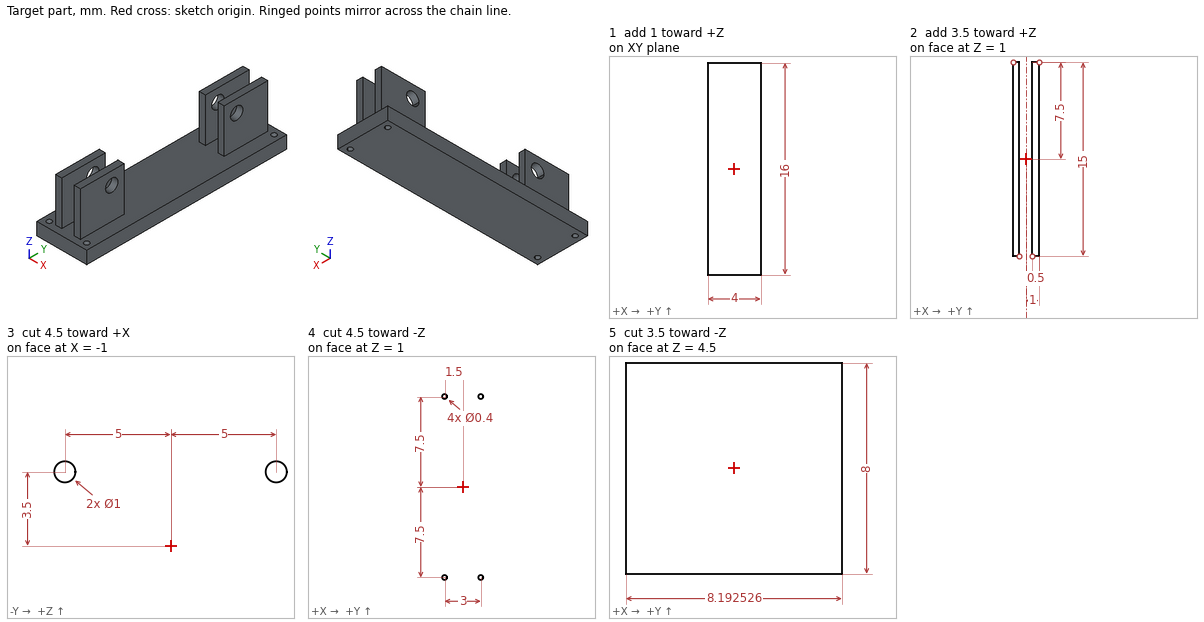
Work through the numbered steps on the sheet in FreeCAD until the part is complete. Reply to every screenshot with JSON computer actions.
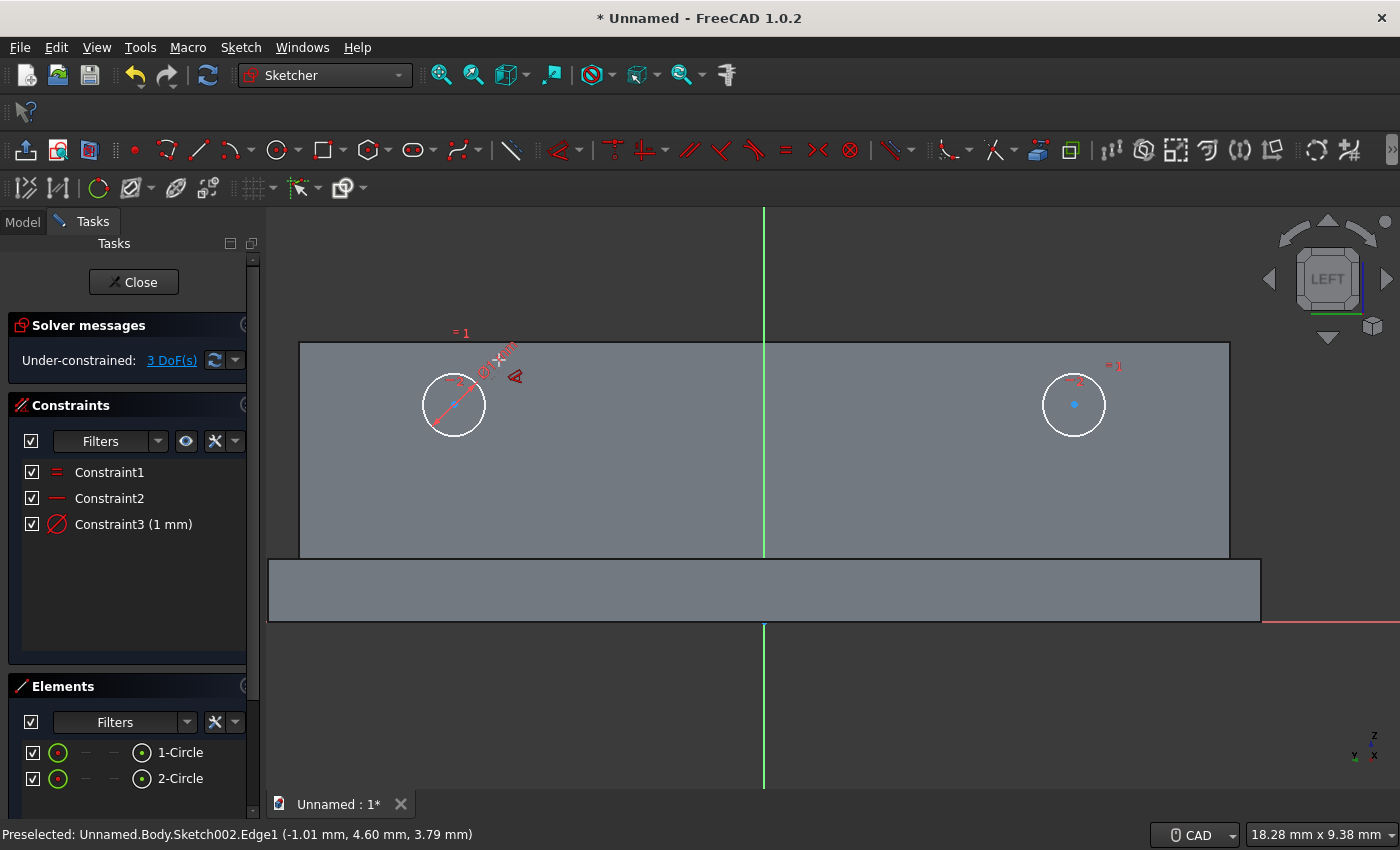
{"action": "left_click", "coordinate": [454, 405]}
{"action": "left_click", "coordinate": [609, 656]}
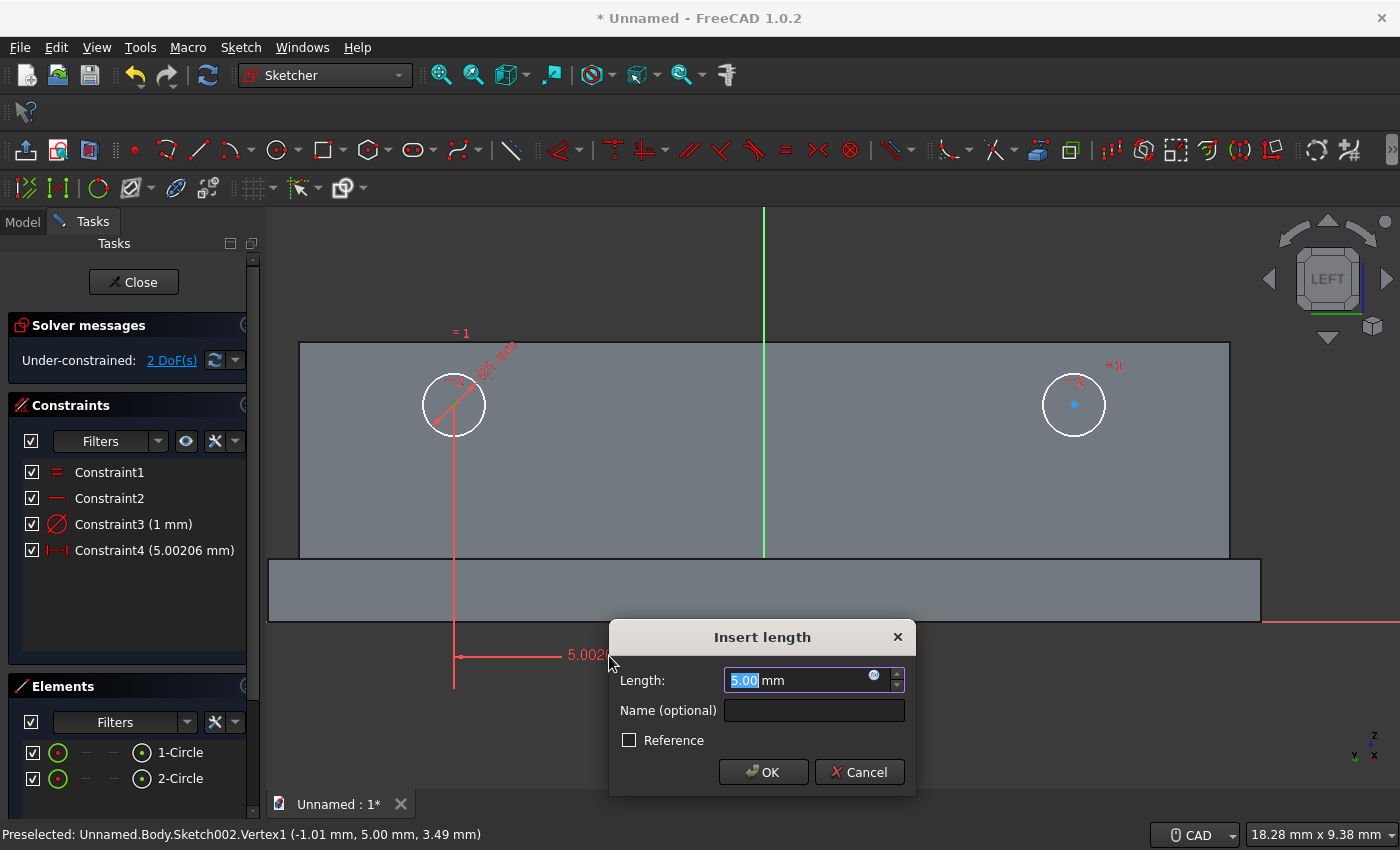
{"action": "type", "text": "5"}
{"action": "key", "text": "Return"}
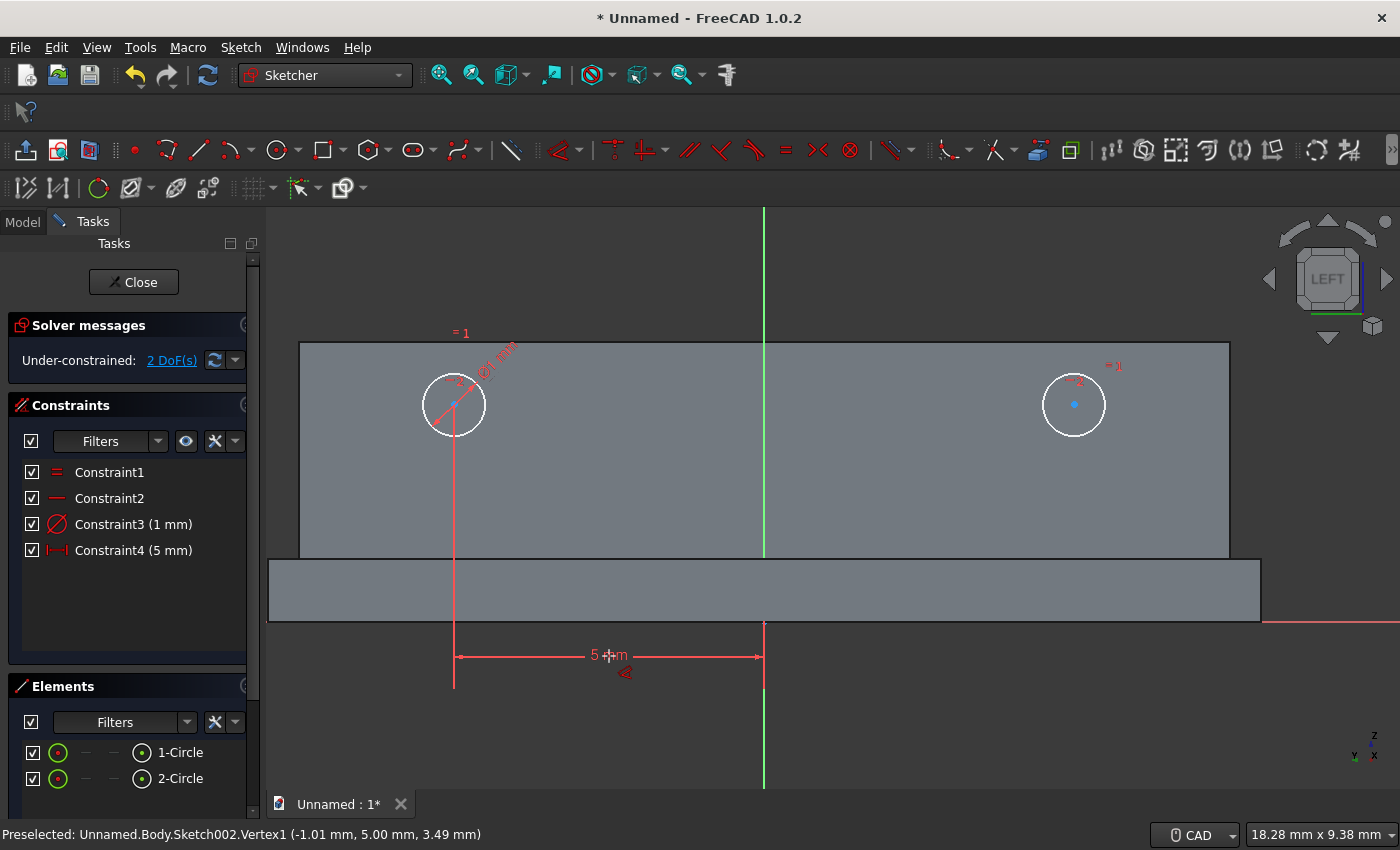
{"action": "left_click", "coordinate": [1074, 405]}
{"action": "left_click", "coordinate": [919, 656]}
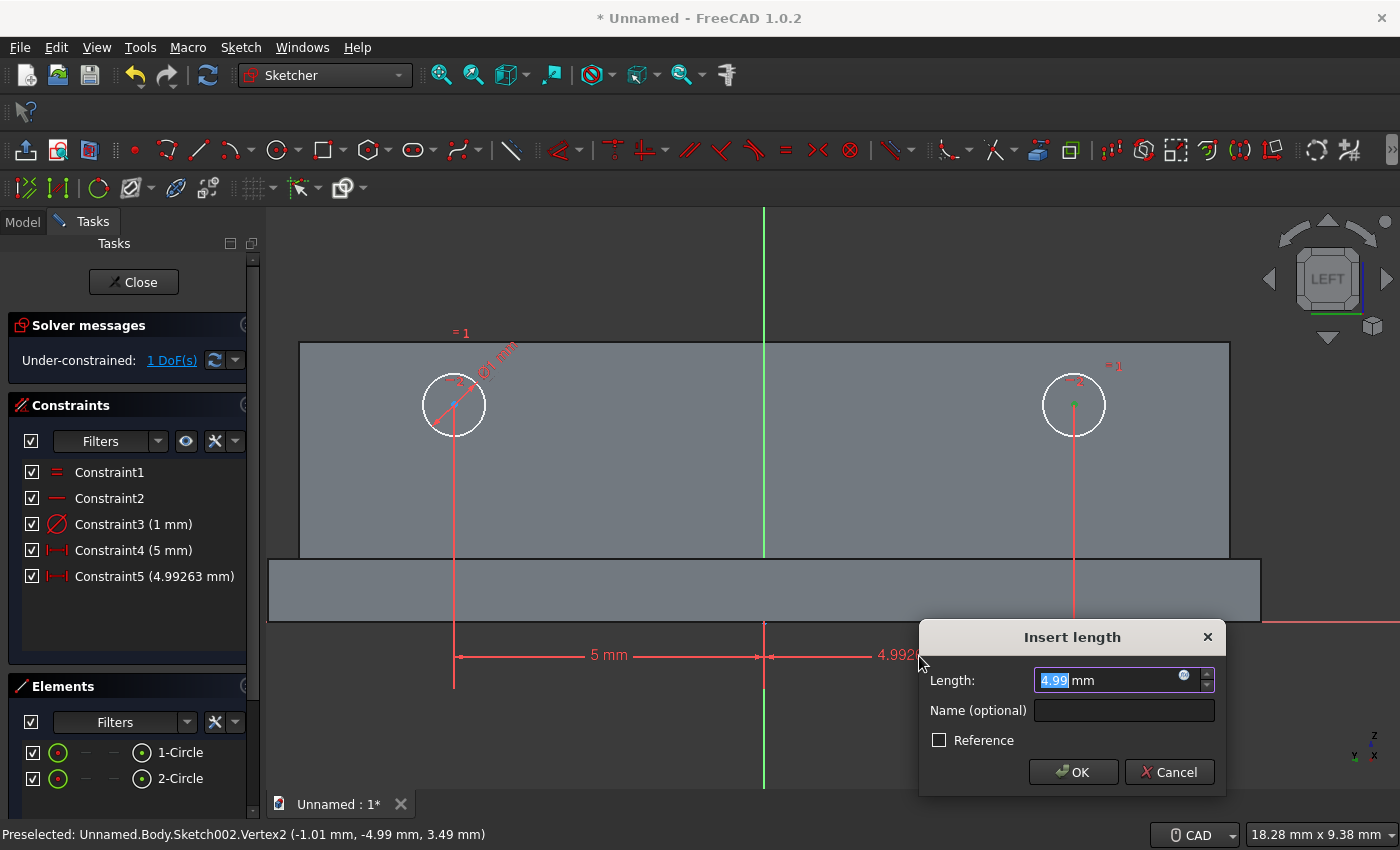
{"action": "type", "text": "5"}
{"action": "key", "text": "Return"}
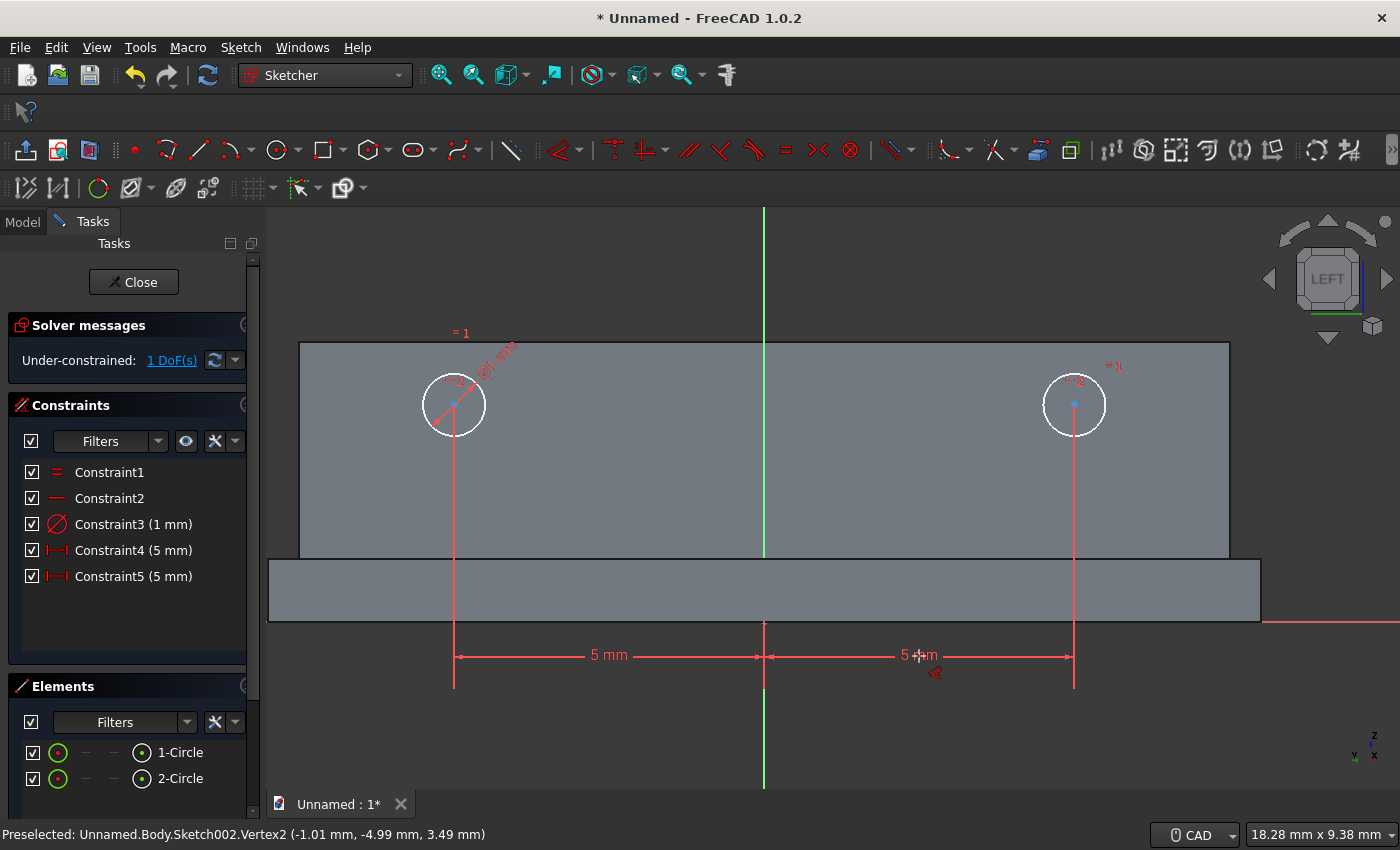
{"action": "left_click", "coordinate": [454, 405]}
{"action": "left_click", "coordinate": [420, 513]}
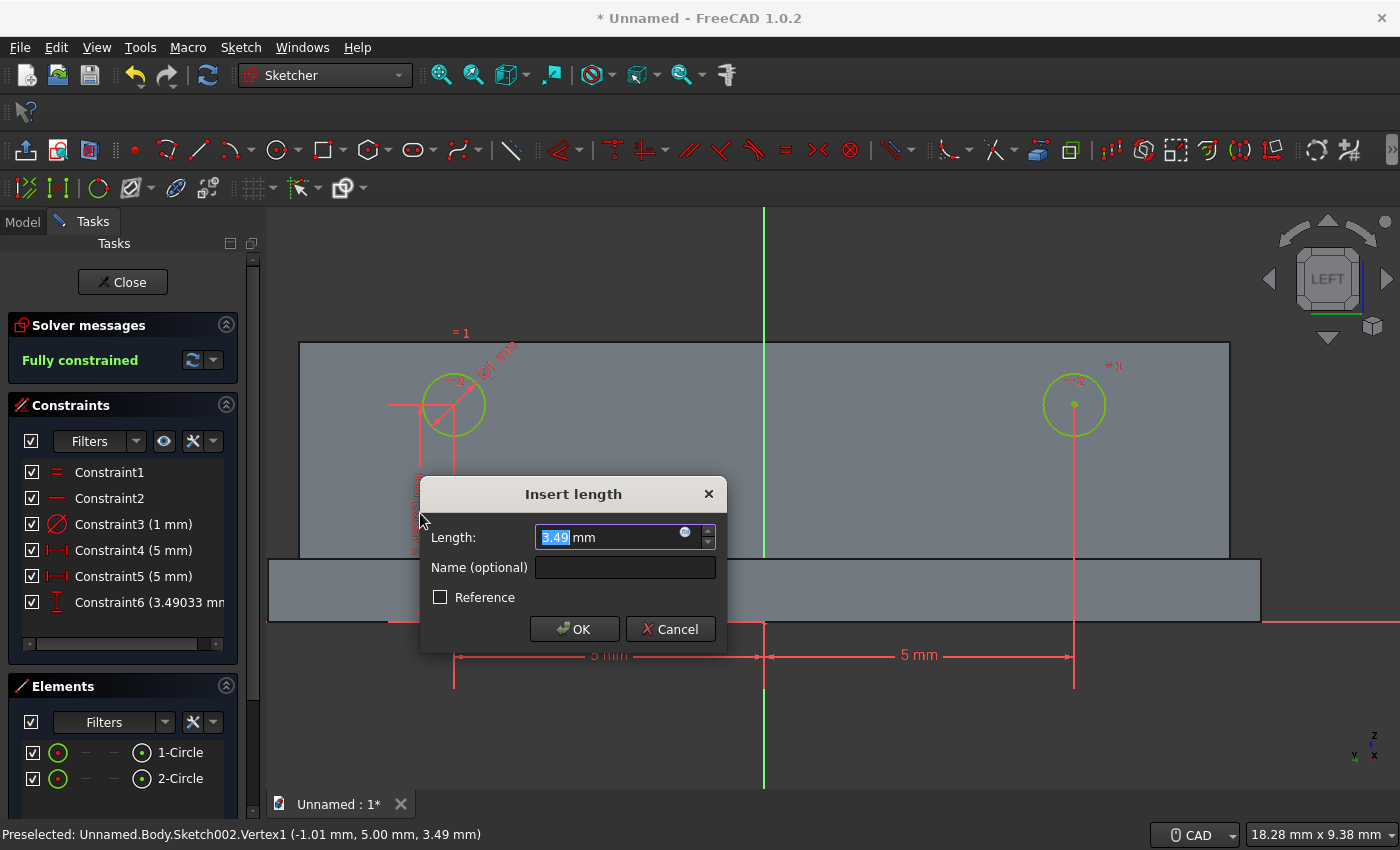
{"action": "type", "text": "3.5"}
{"action": "key", "text": "Return"}
{"action": "key", "text": "Escape"}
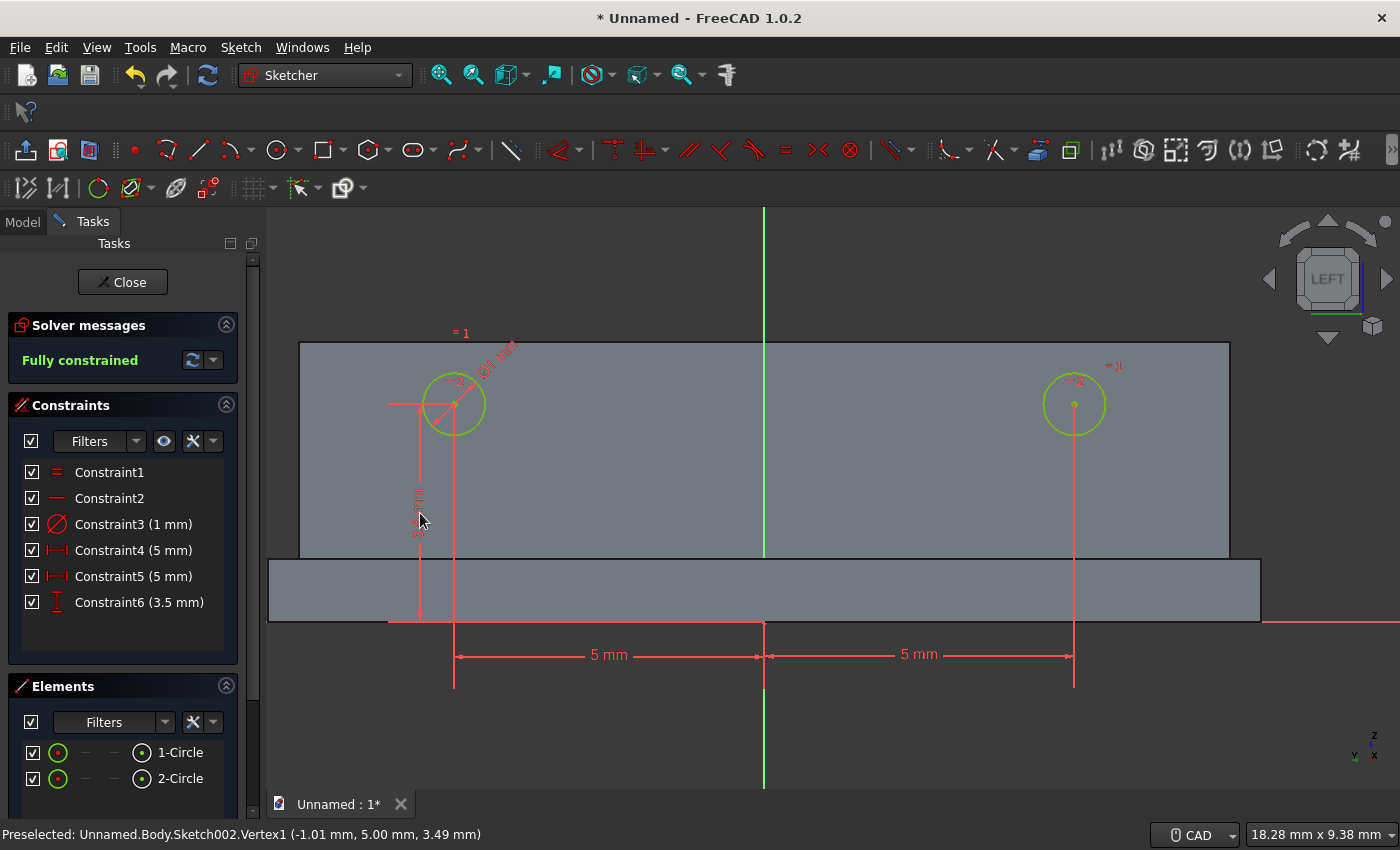
{"action": "left_click", "coordinate": [123, 282]}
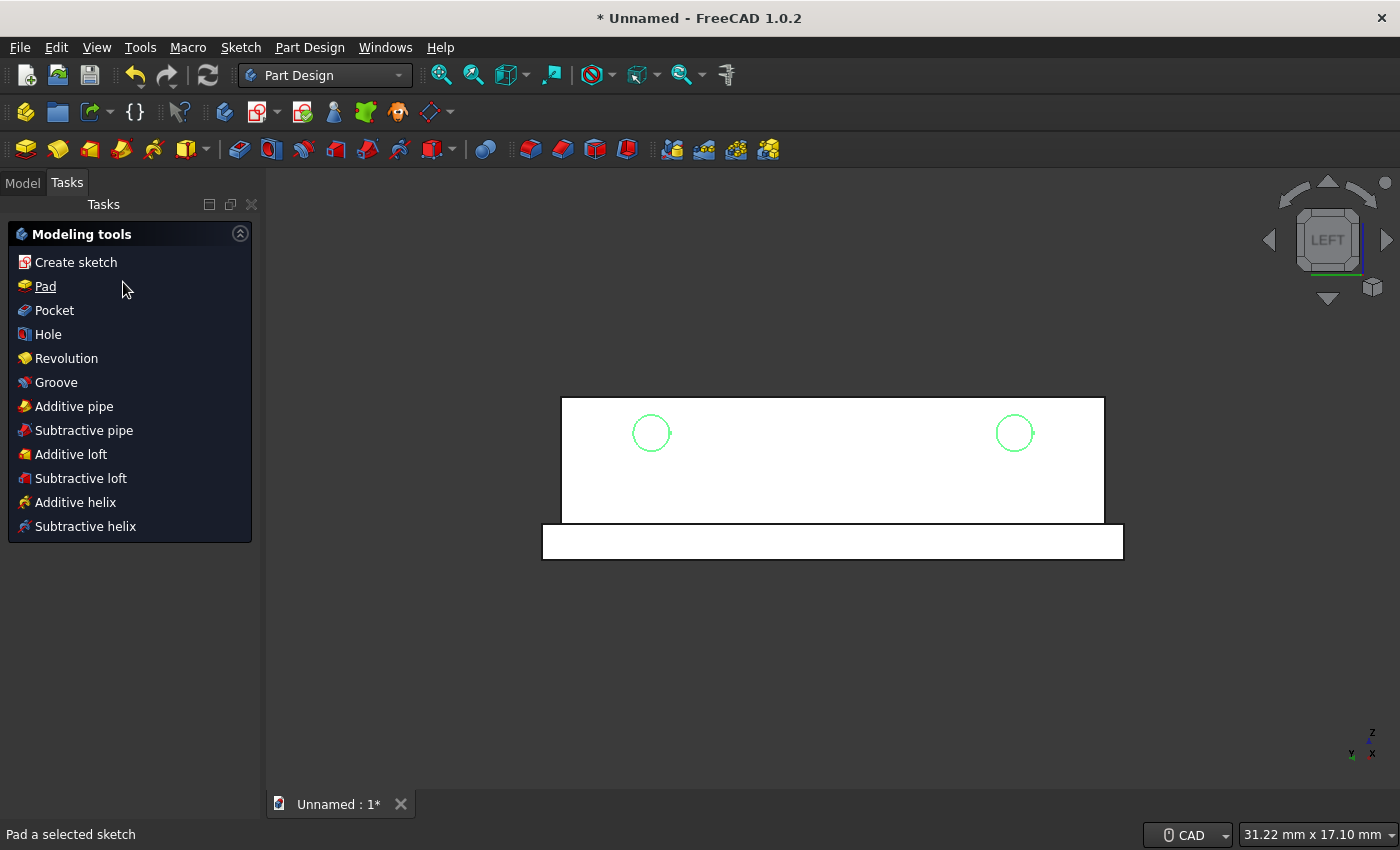
{"action": "left_click", "coordinate": [240, 150]}